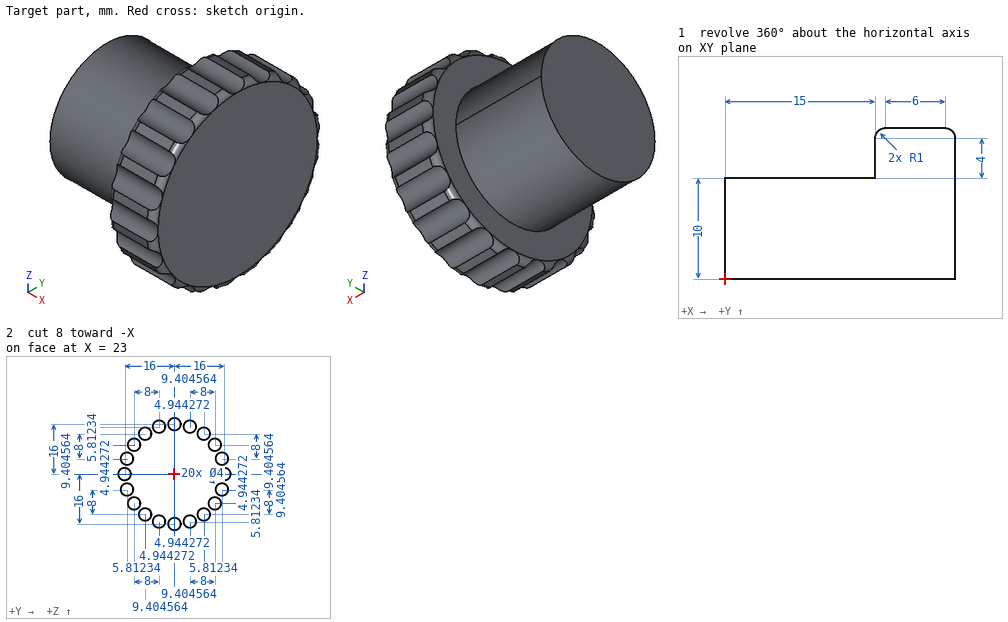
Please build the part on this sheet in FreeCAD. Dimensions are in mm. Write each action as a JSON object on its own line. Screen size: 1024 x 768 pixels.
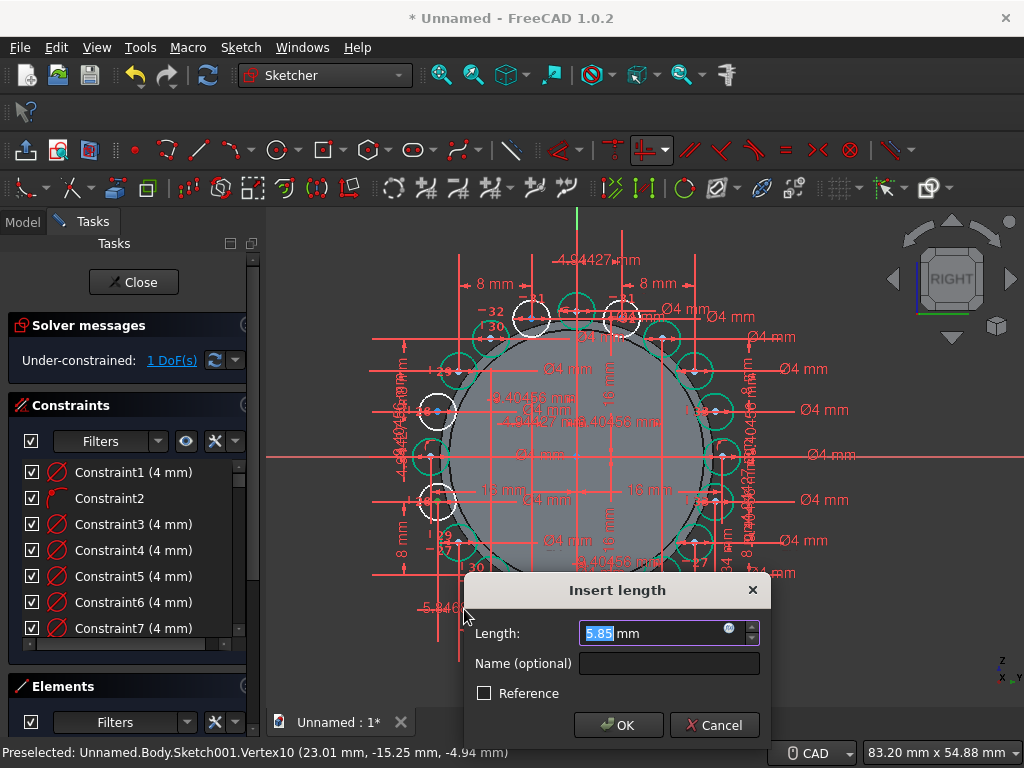
{"action": "type", "text": "5.81234"}
{"action": "key", "text": "Return"}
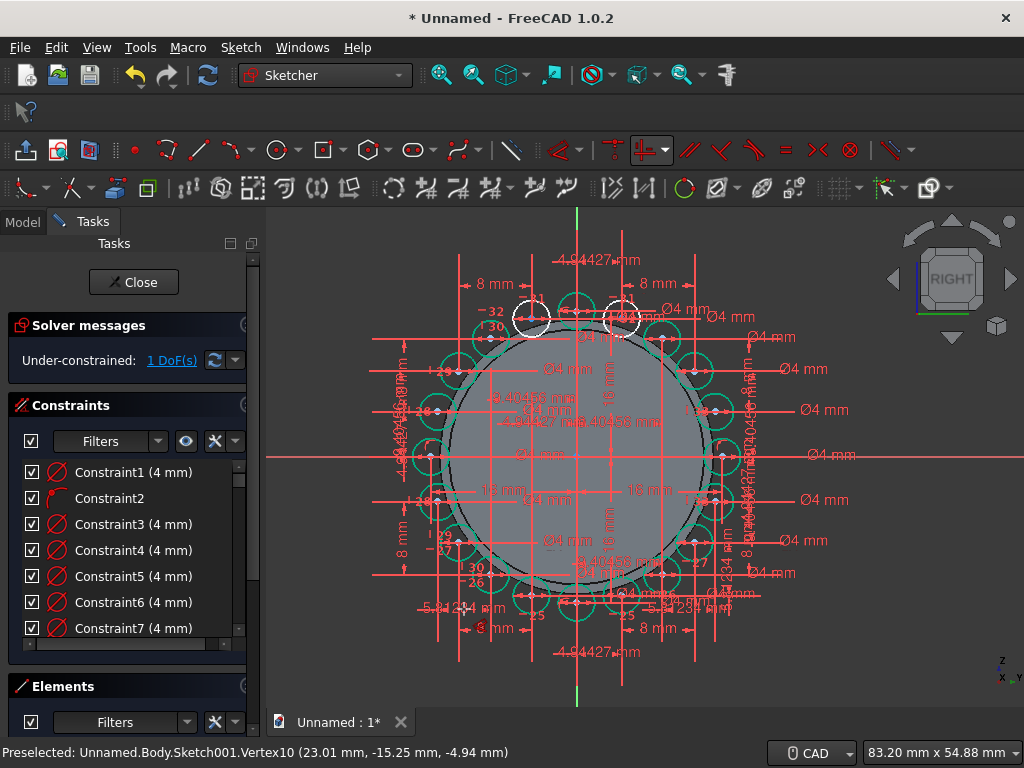
{"action": "left_click", "coordinate": [459, 371]}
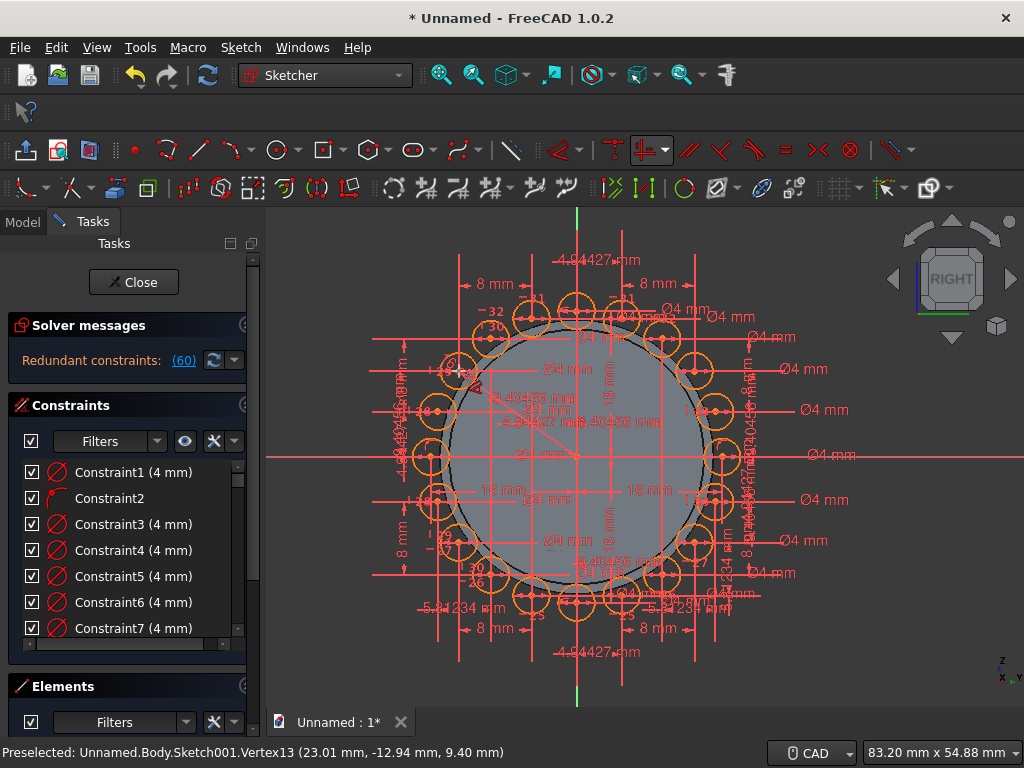
{"action": "left_click", "coordinate": [532, 319]}
{"action": "left_click", "coordinate": [425, 345]}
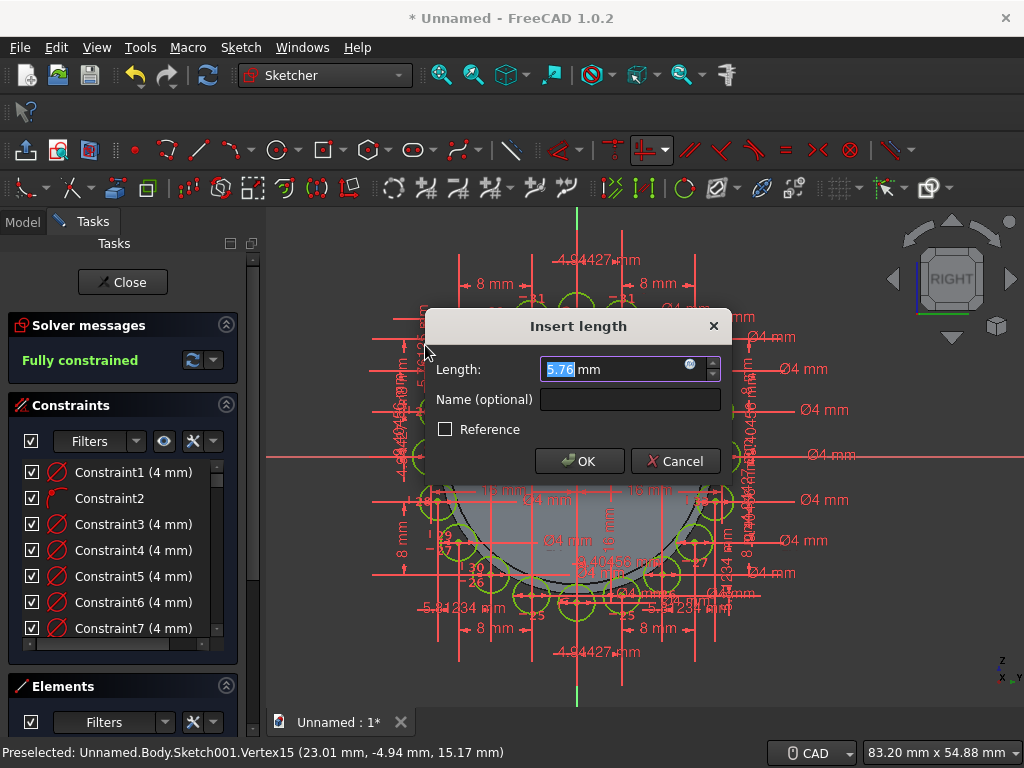
{"action": "type", "text": "5.81234"}
{"action": "key", "text": "Return"}
{"action": "key", "text": "Escape"}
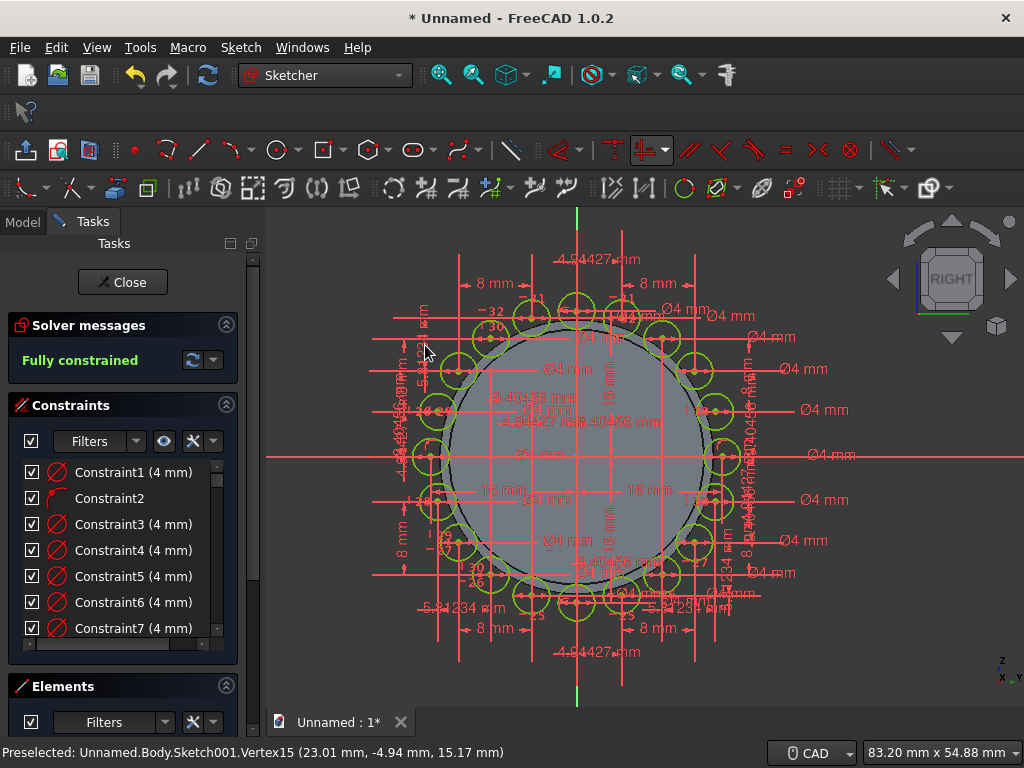
{"action": "left_click", "coordinate": [123, 282]}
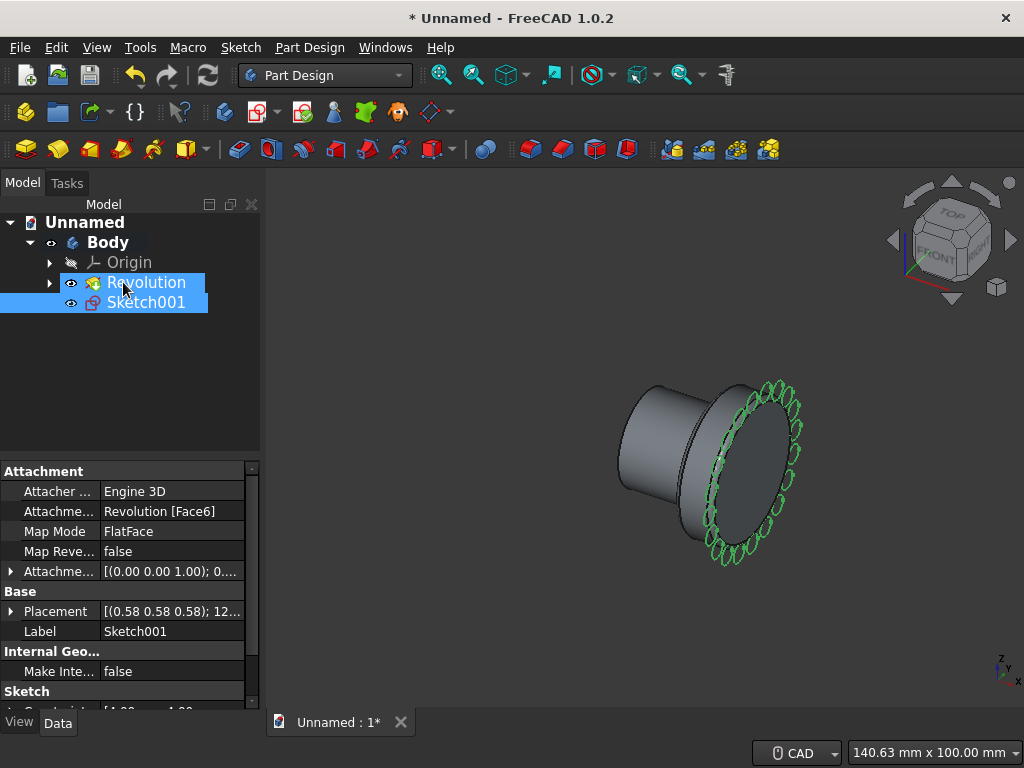
{"action": "left_click", "coordinate": [240, 150]}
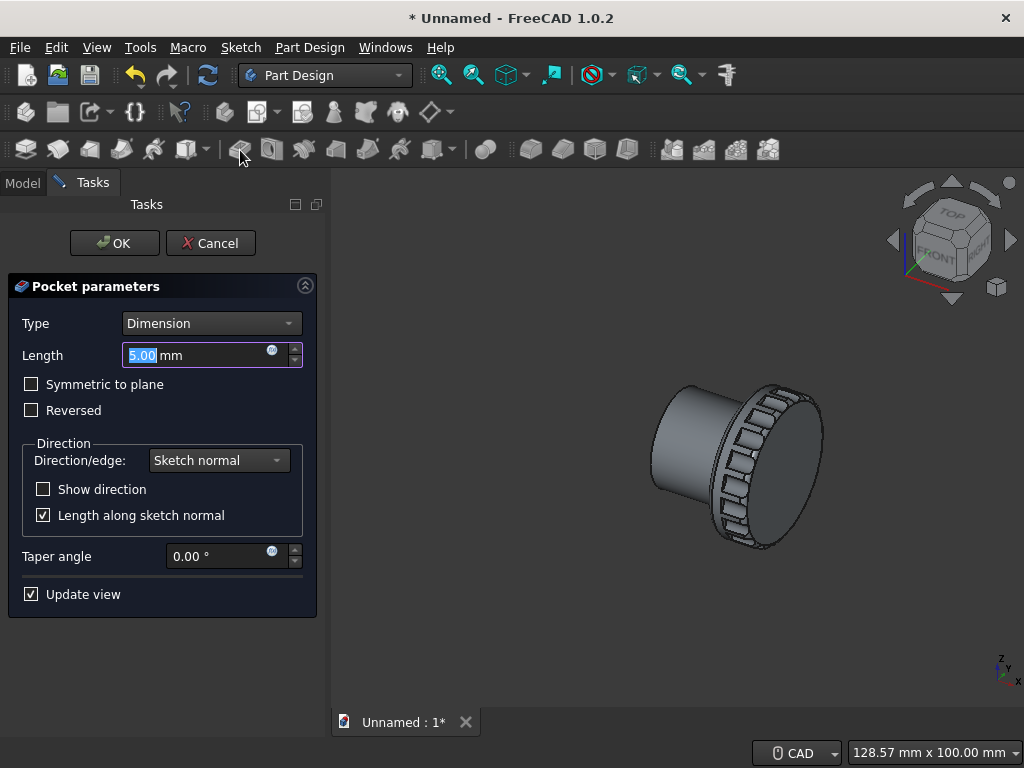
{"action": "type", "text": "8"}
{"action": "key", "text": "Tab"}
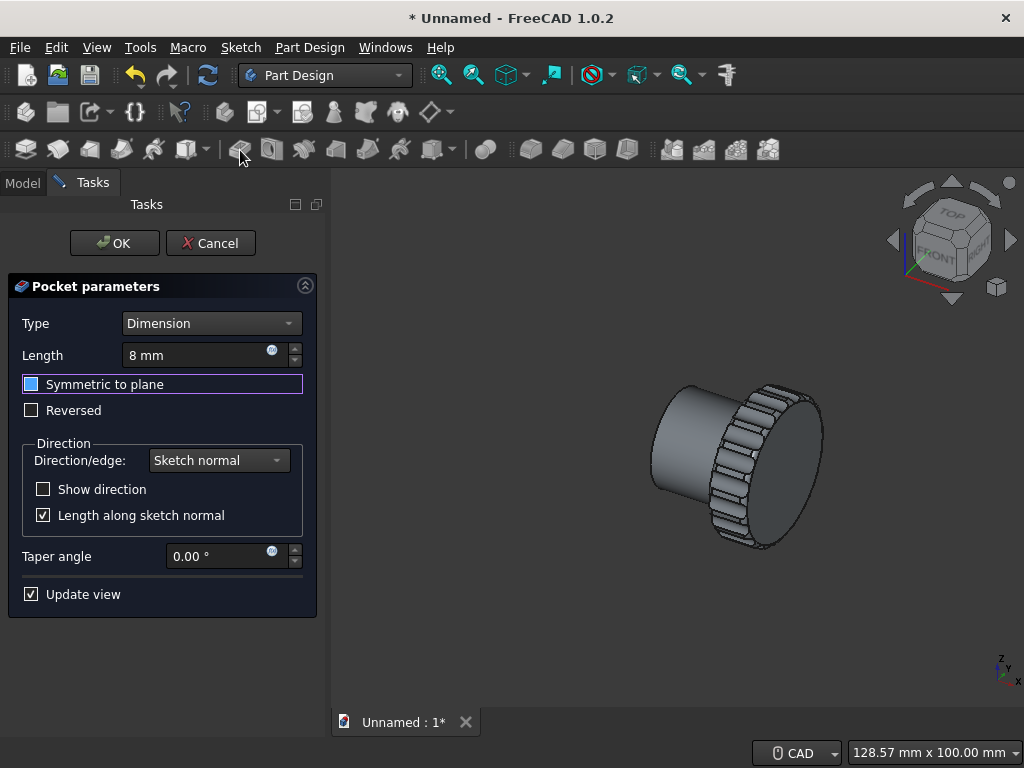
{"action": "left_click", "coordinate": [115, 243]}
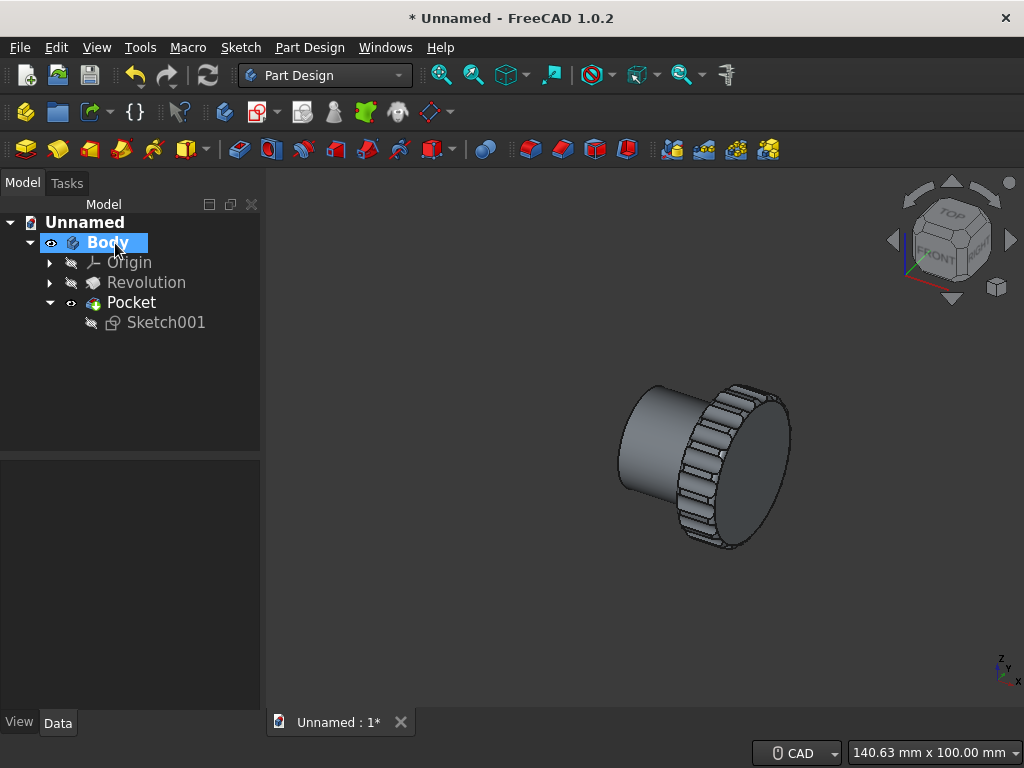
{"action": "key", "text": "0"}